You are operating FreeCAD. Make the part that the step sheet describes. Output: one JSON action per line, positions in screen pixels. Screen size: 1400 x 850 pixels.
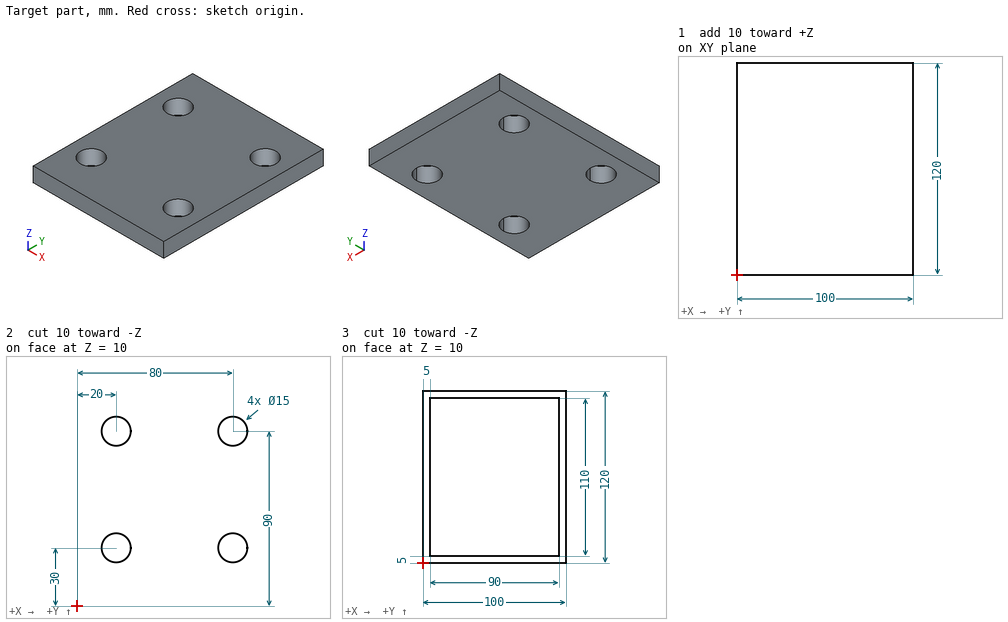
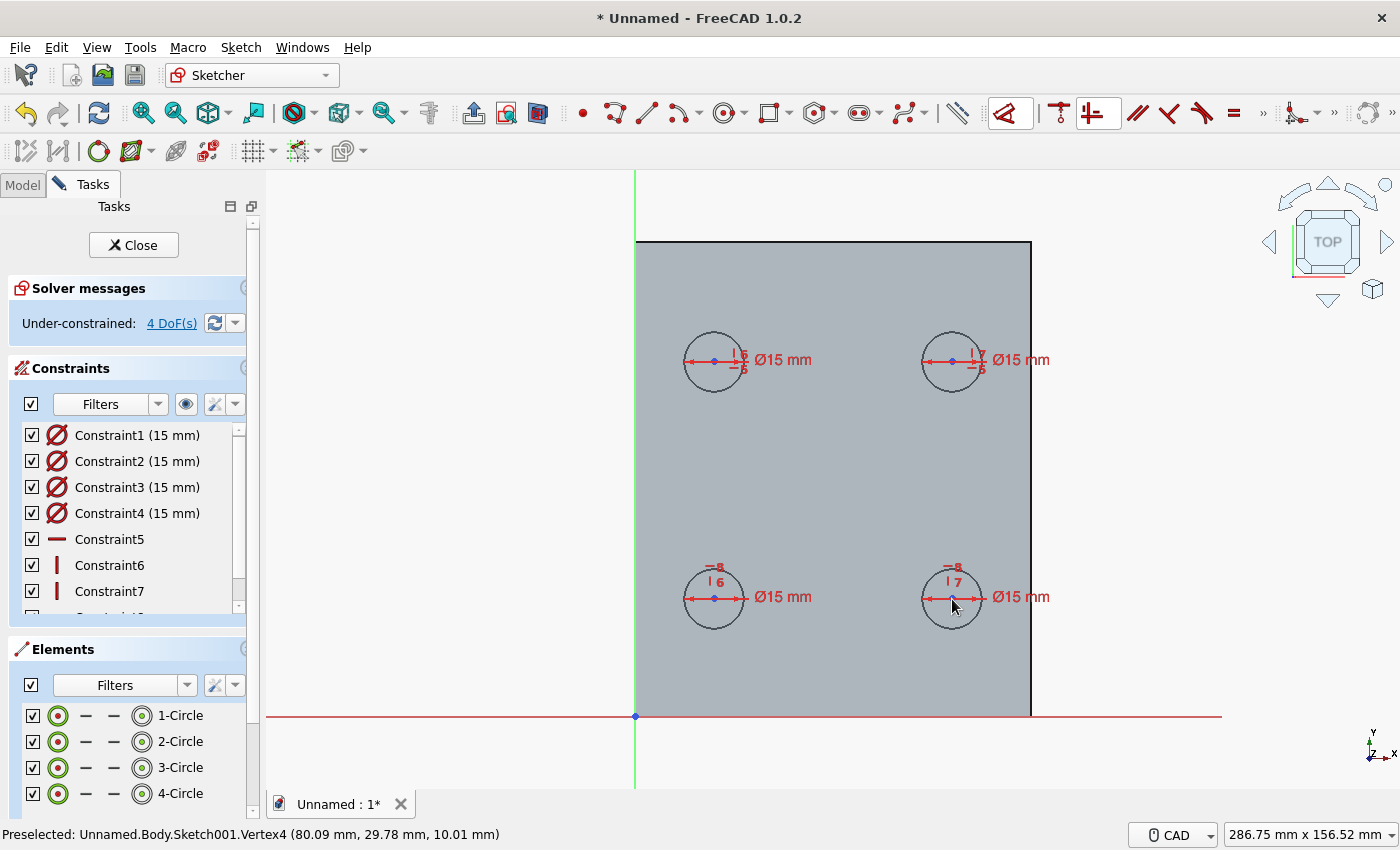
{"action": "key", "text": "d"}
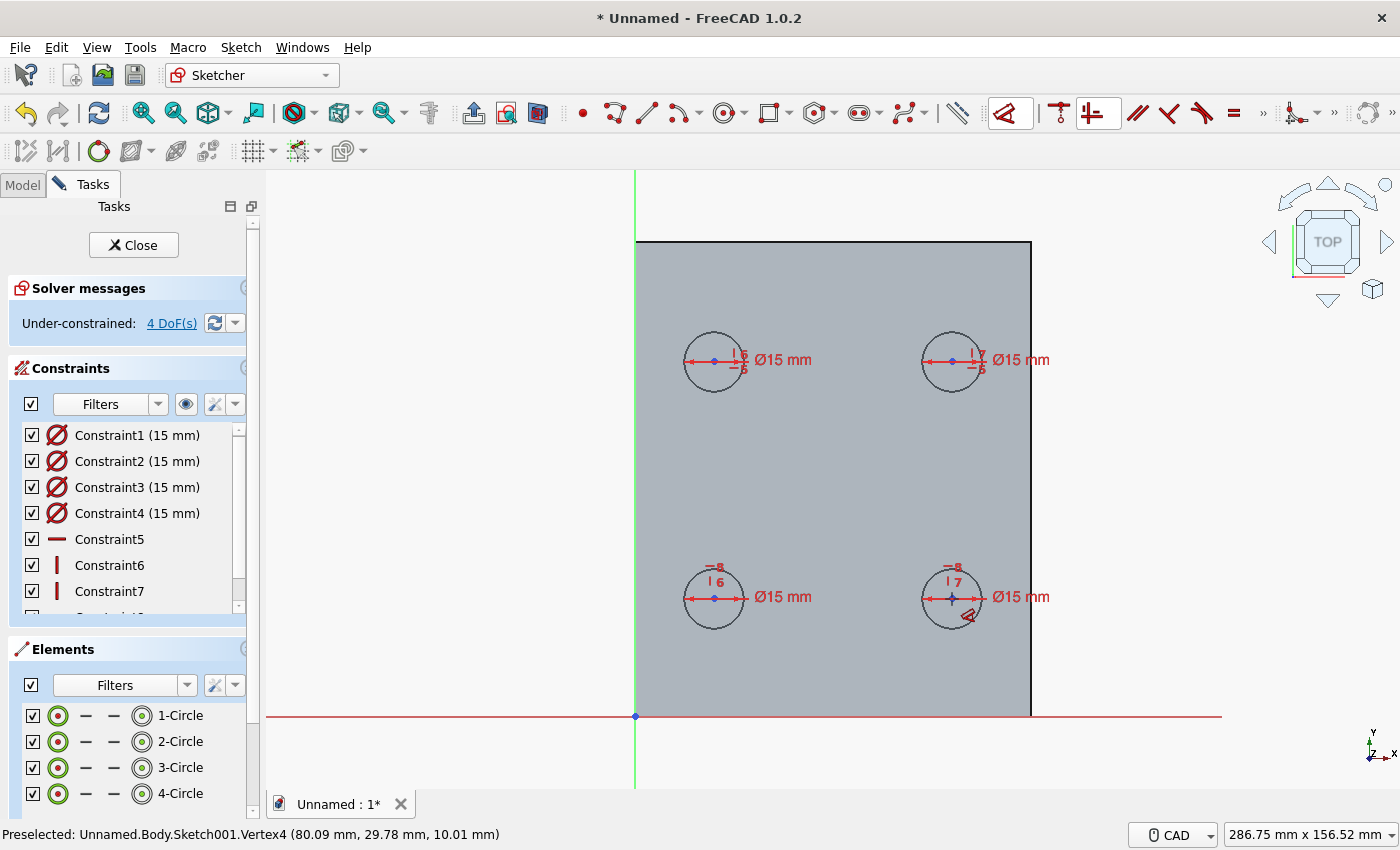
{"action": "left_click", "coordinate": [952, 362]}
{"action": "left_click", "coordinate": [794, 751]}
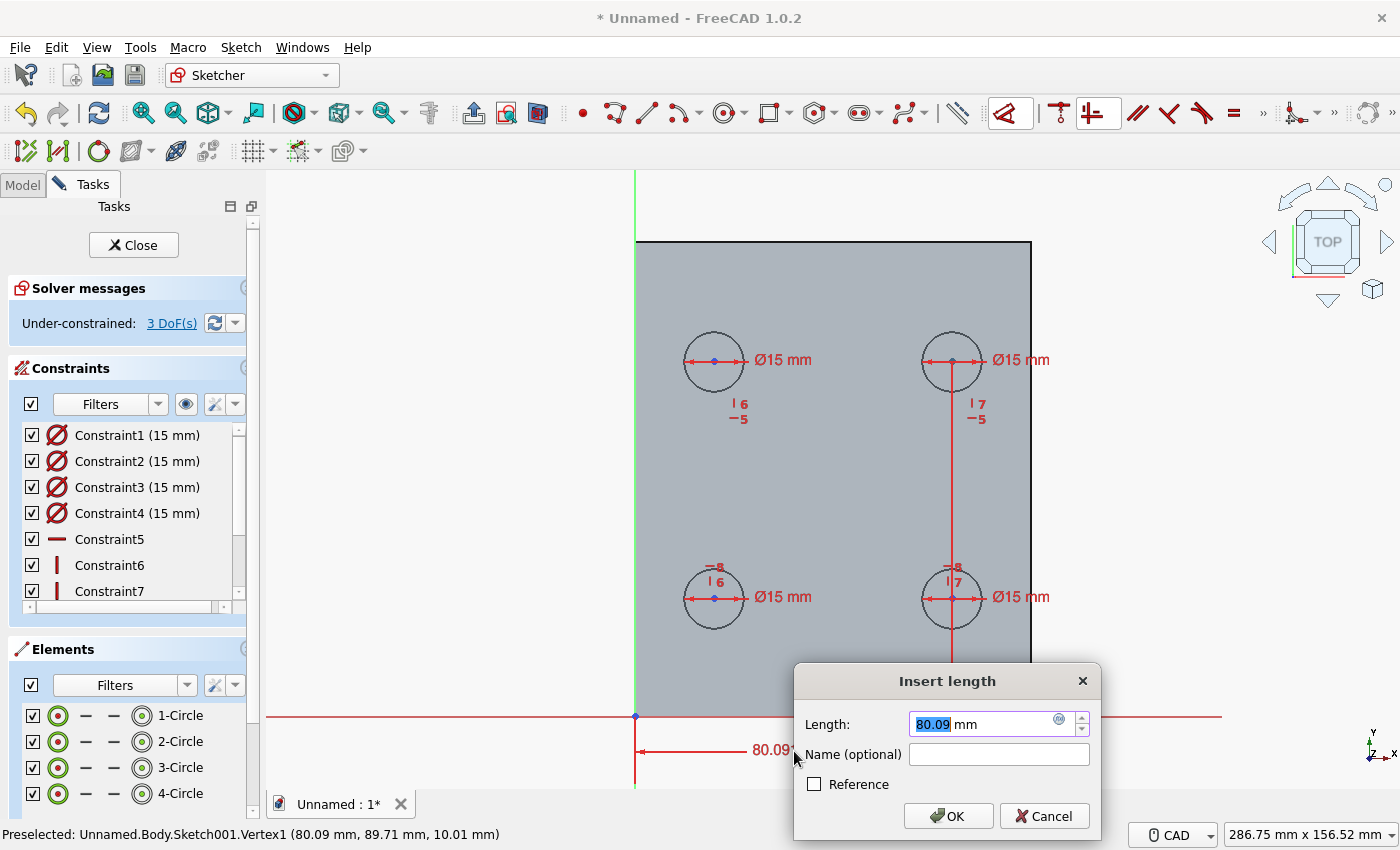
{"action": "type", "text": "80"}
{"action": "key", "text": "Return"}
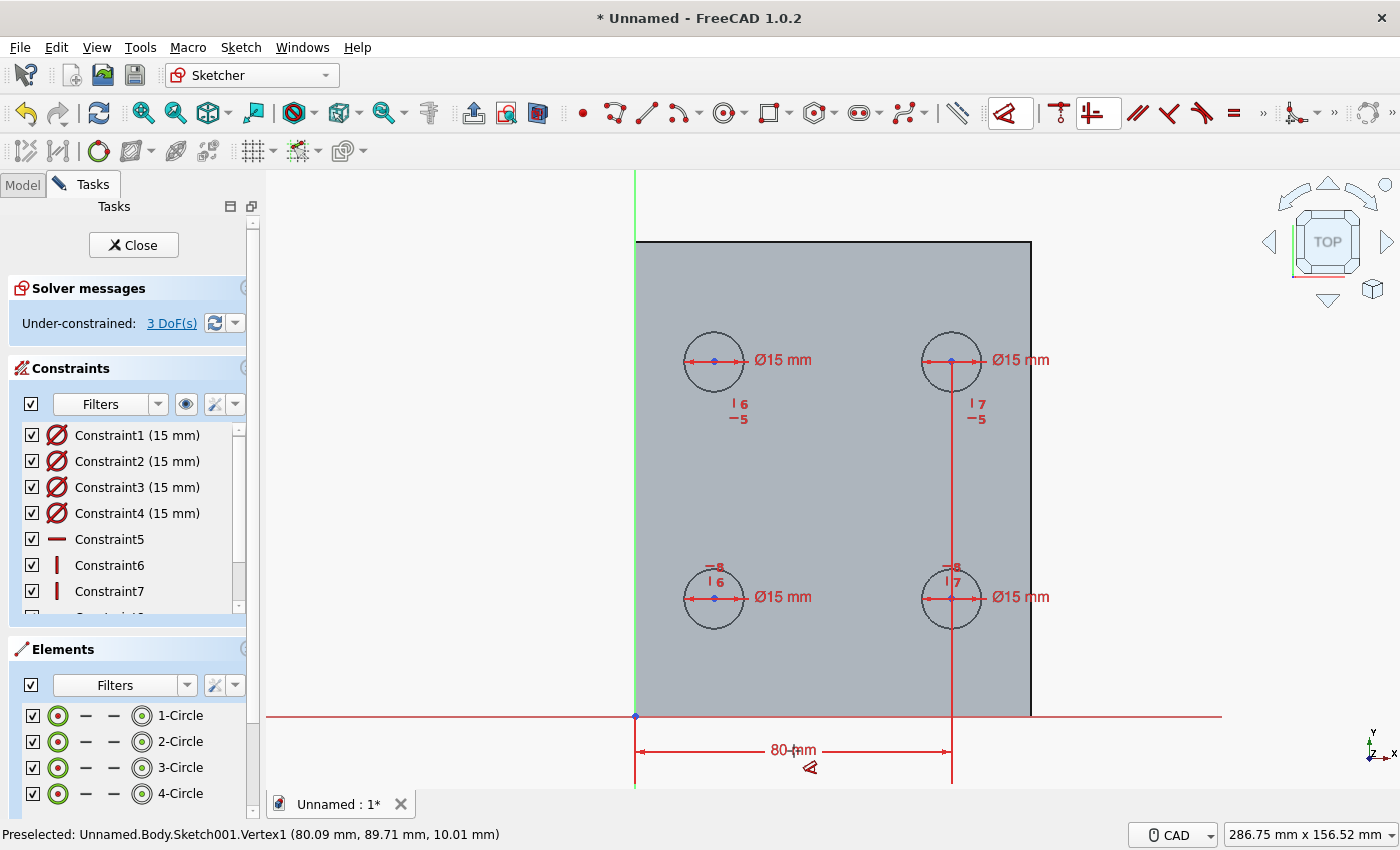
{"action": "left_click", "coordinate": [952, 362]}
{"action": "left_click", "coordinate": [601, 539]}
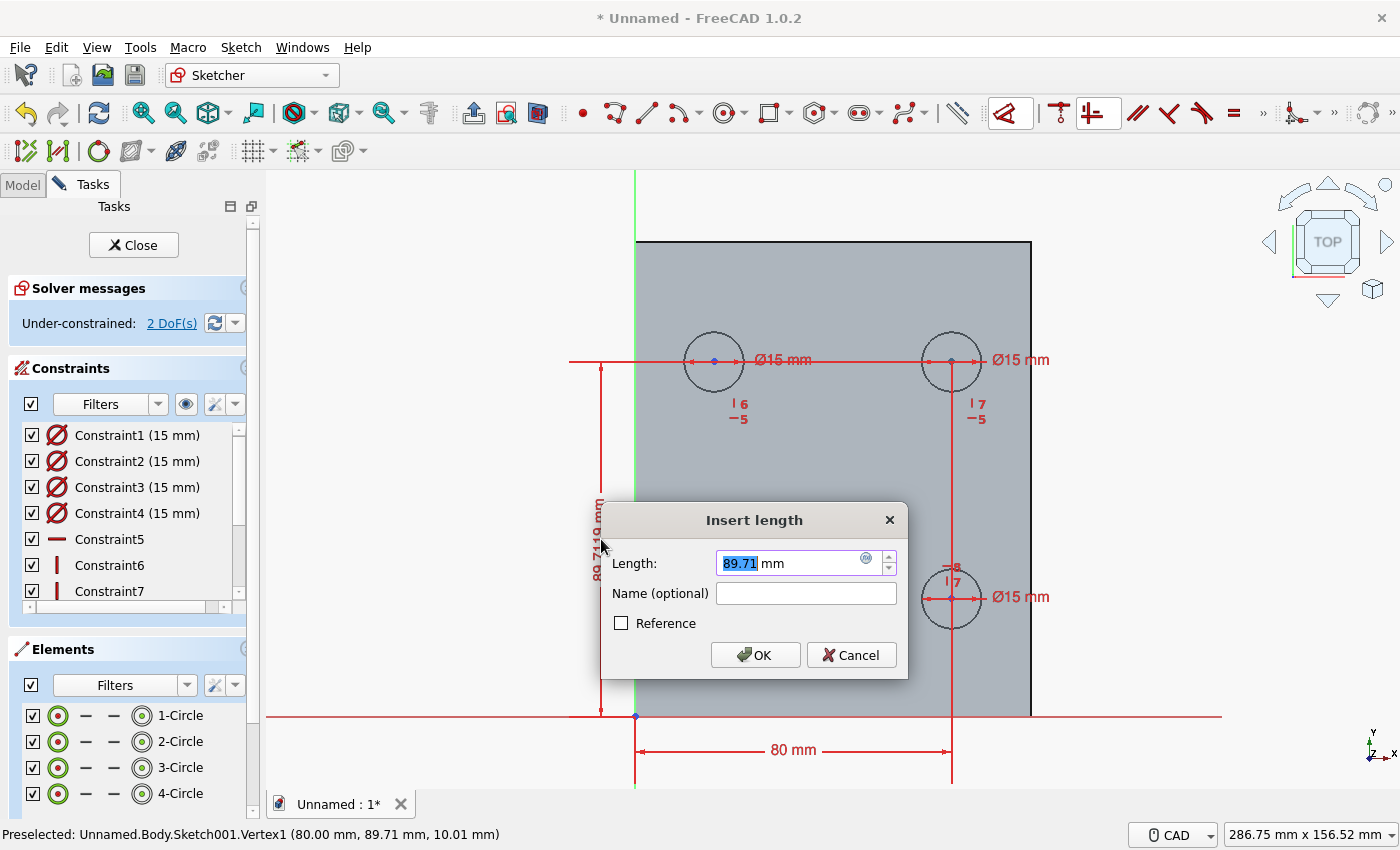
{"action": "type", "text": "90"}
{"action": "key", "text": "Return"}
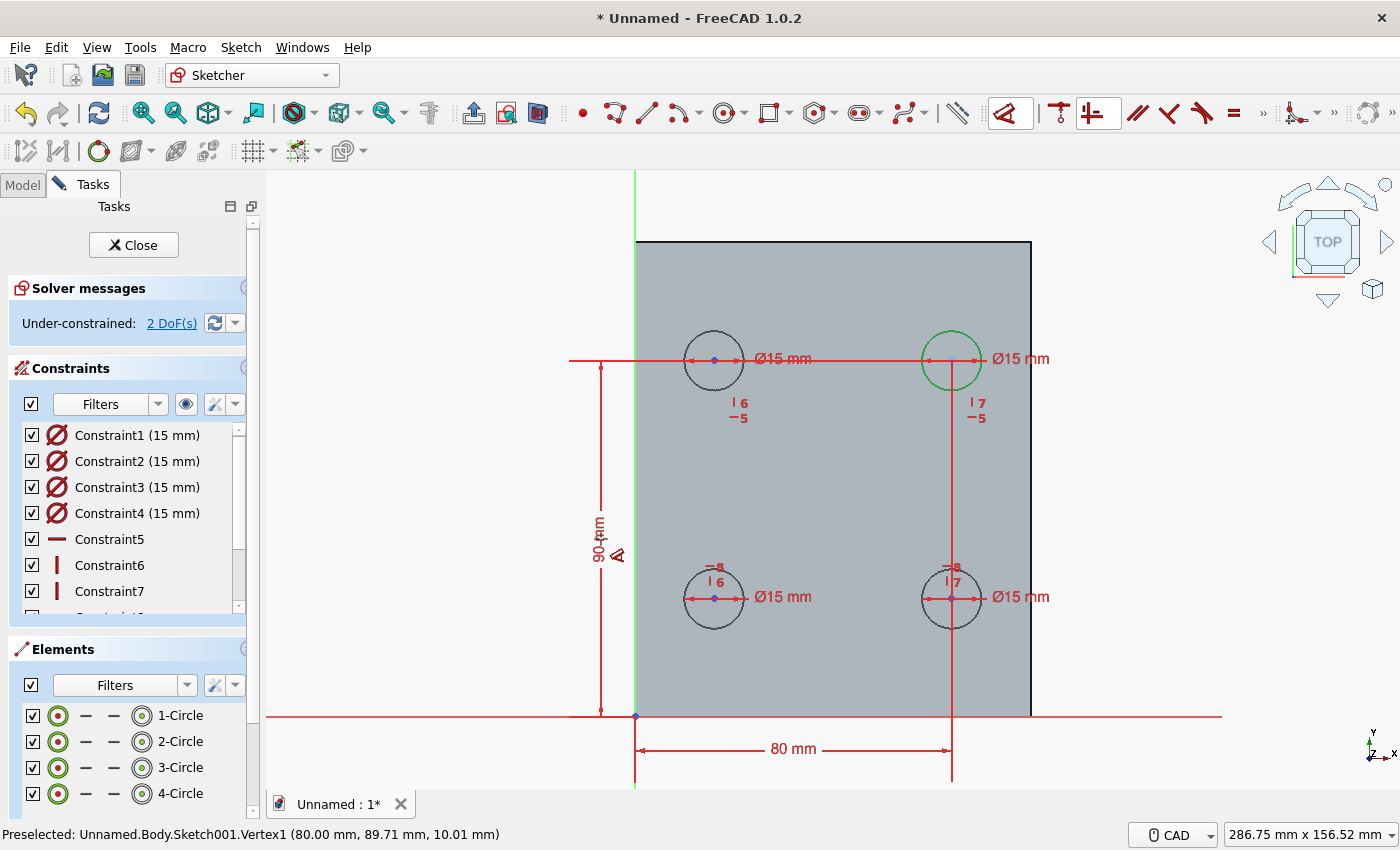
{"action": "left_click", "coordinate": [714, 361]}
{"action": "left_click", "coordinate": [675, 751]}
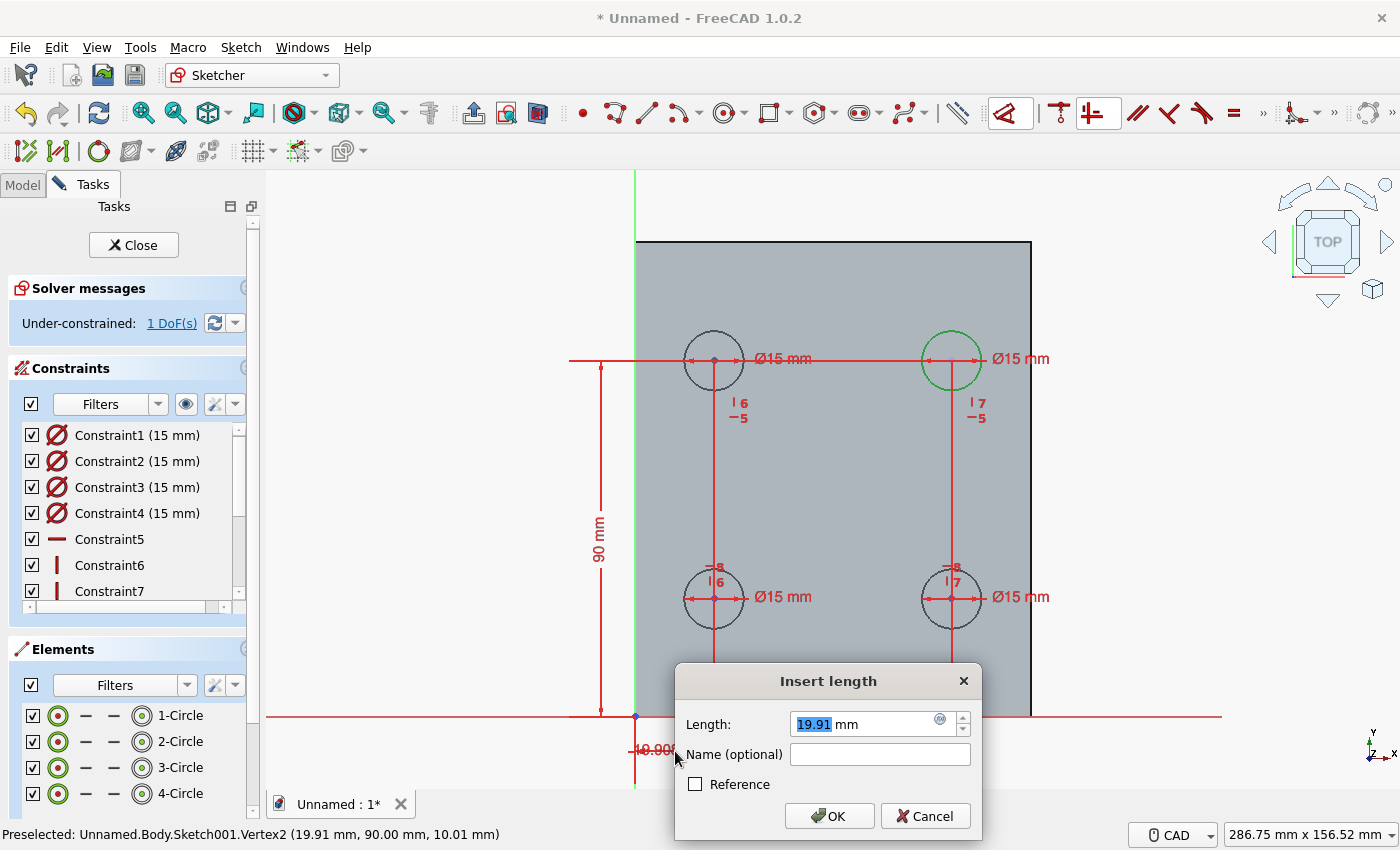
{"action": "type", "text": "20"}
{"action": "key", "text": "Return"}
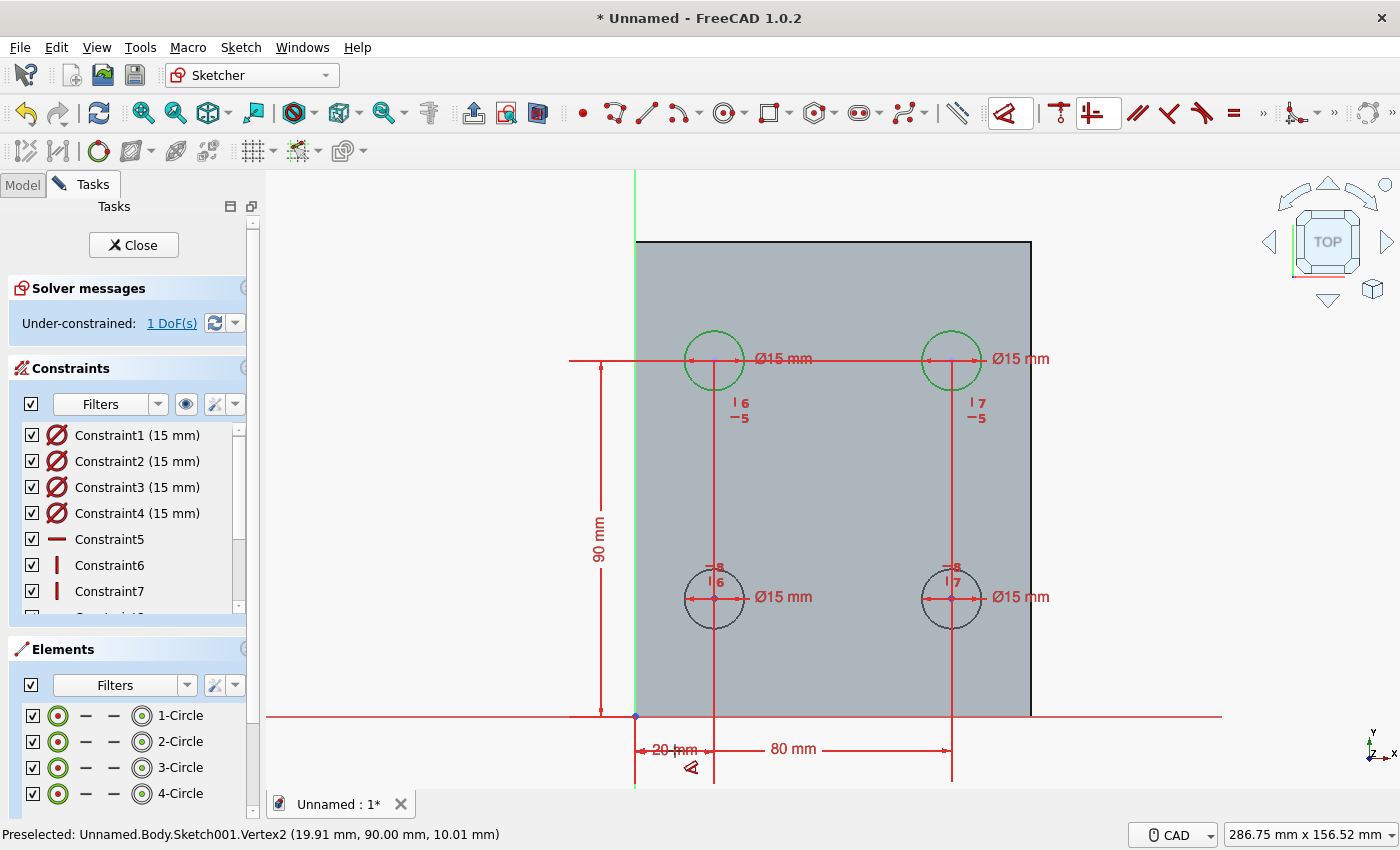
{"action": "left_click", "coordinate": [714, 599]}
{"action": "left_click", "coordinate": [601, 658]}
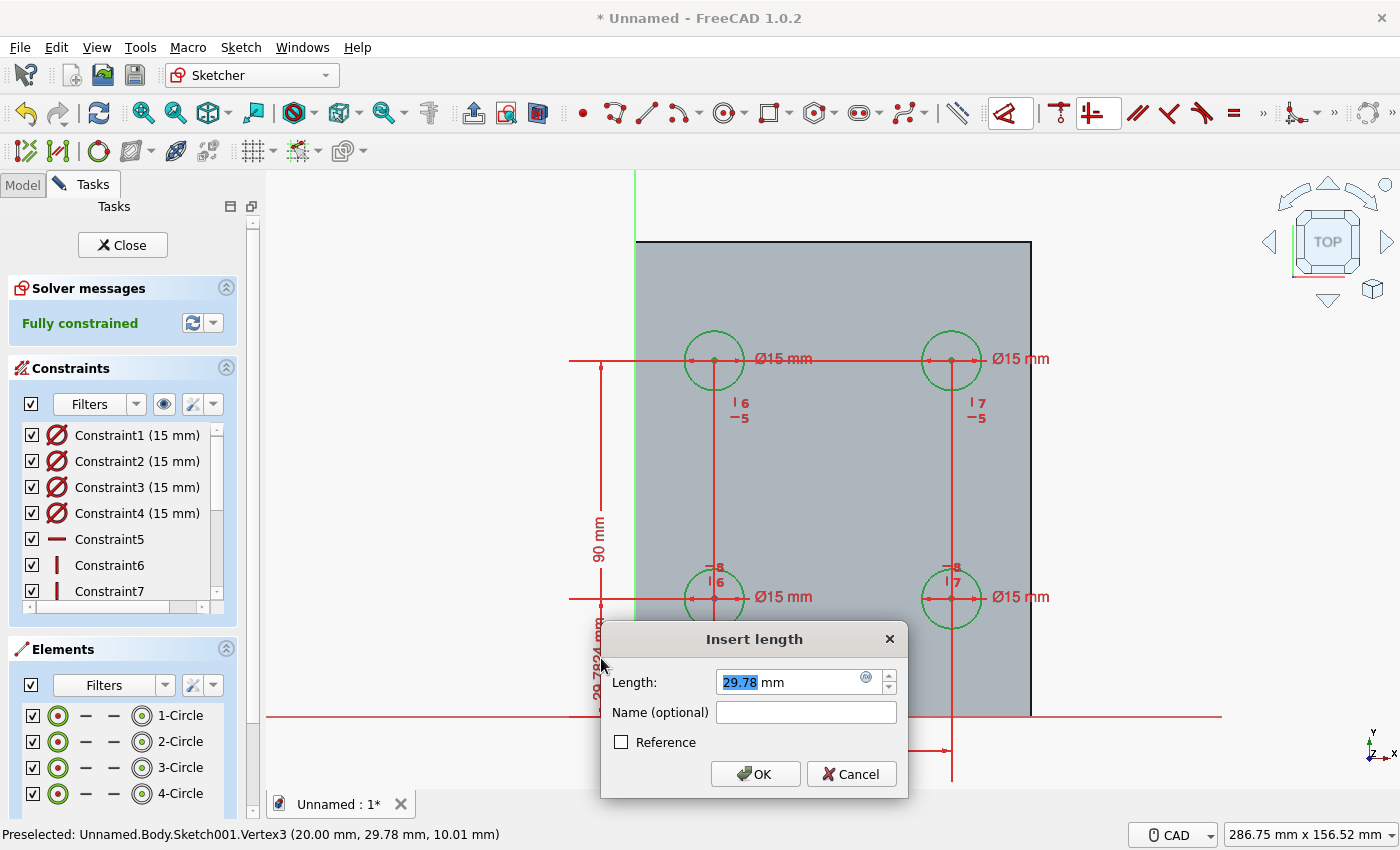
{"action": "type", "text": "30"}
{"action": "key", "text": "Return"}
{"action": "key", "text": "Escape"}